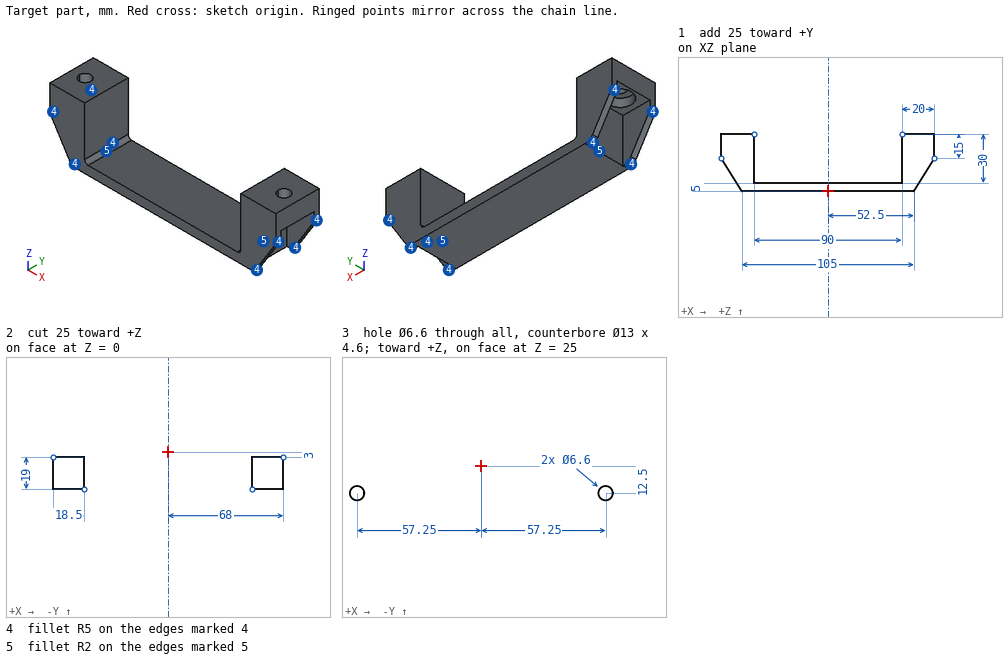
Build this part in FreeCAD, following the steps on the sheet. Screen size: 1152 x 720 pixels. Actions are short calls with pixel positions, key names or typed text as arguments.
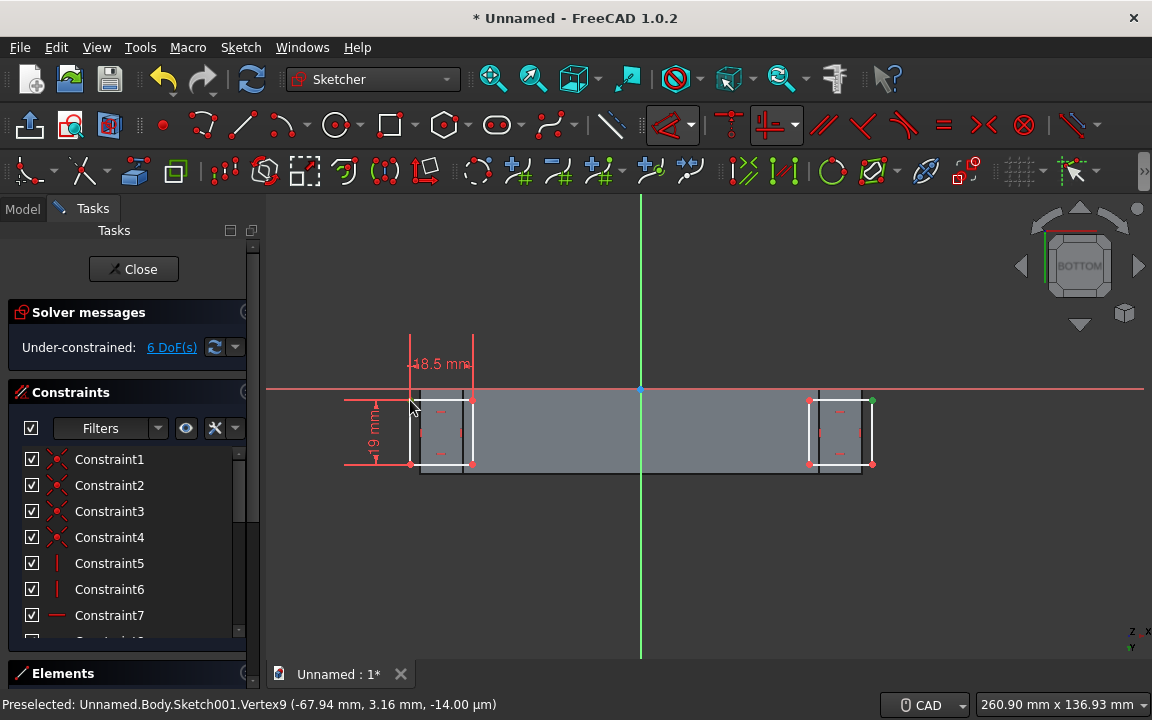
click(641, 602)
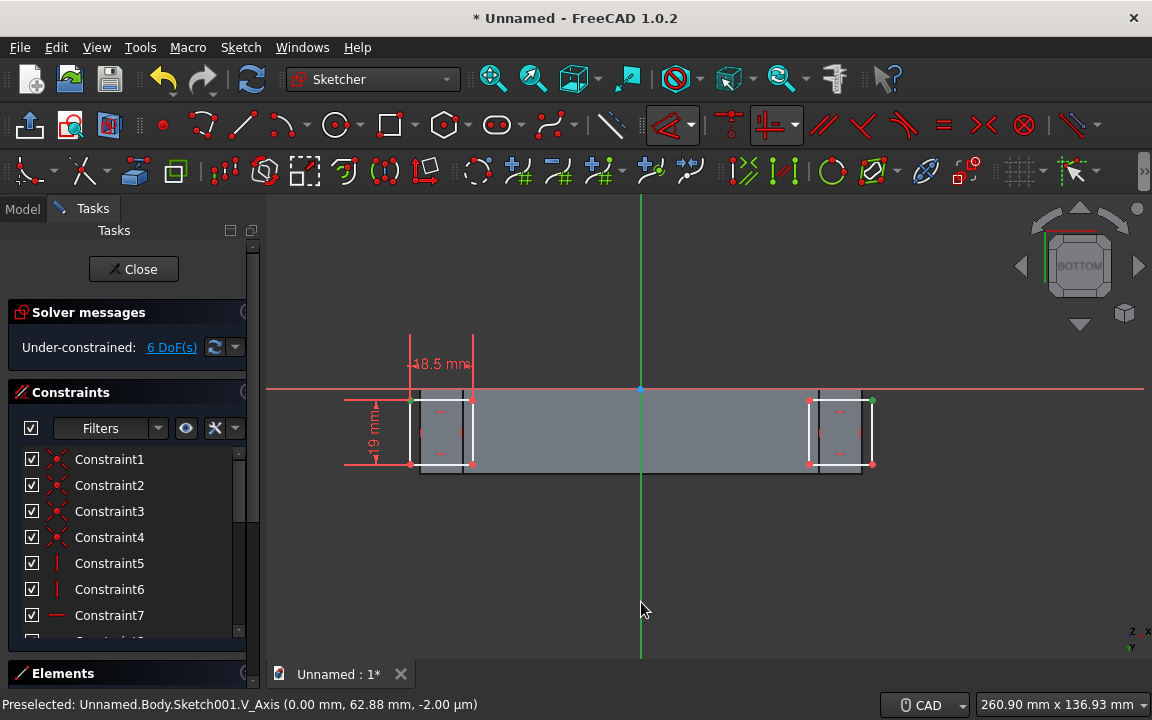
click(984, 126)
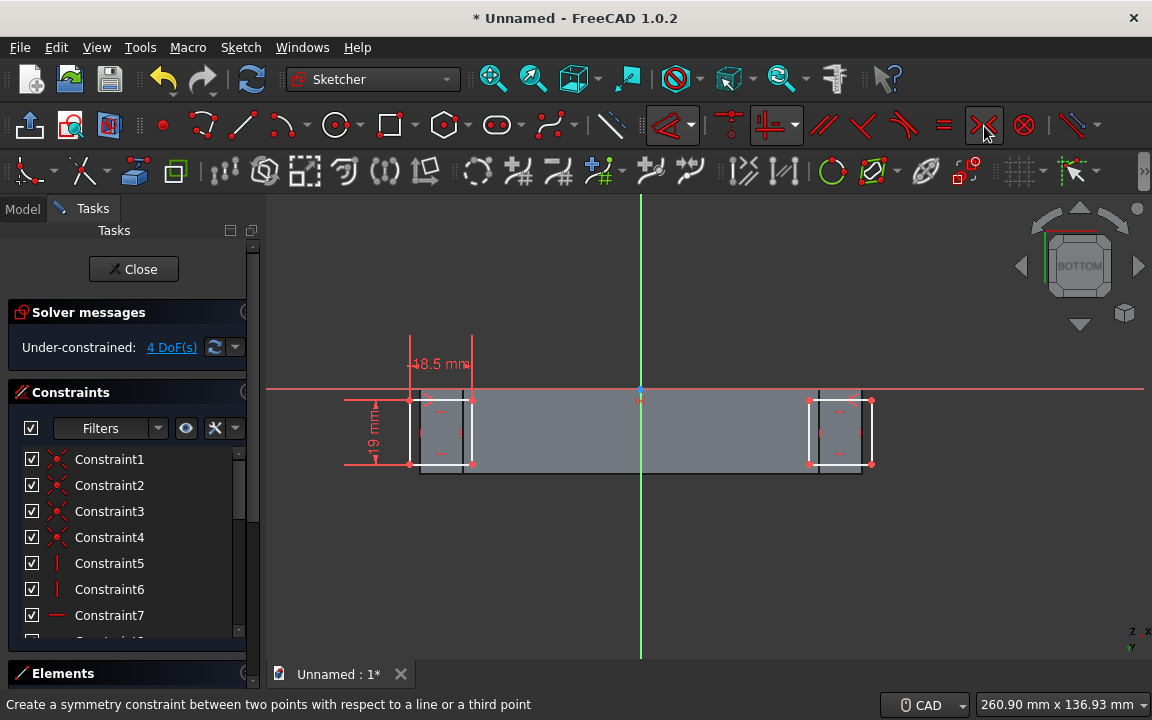
click(809, 465)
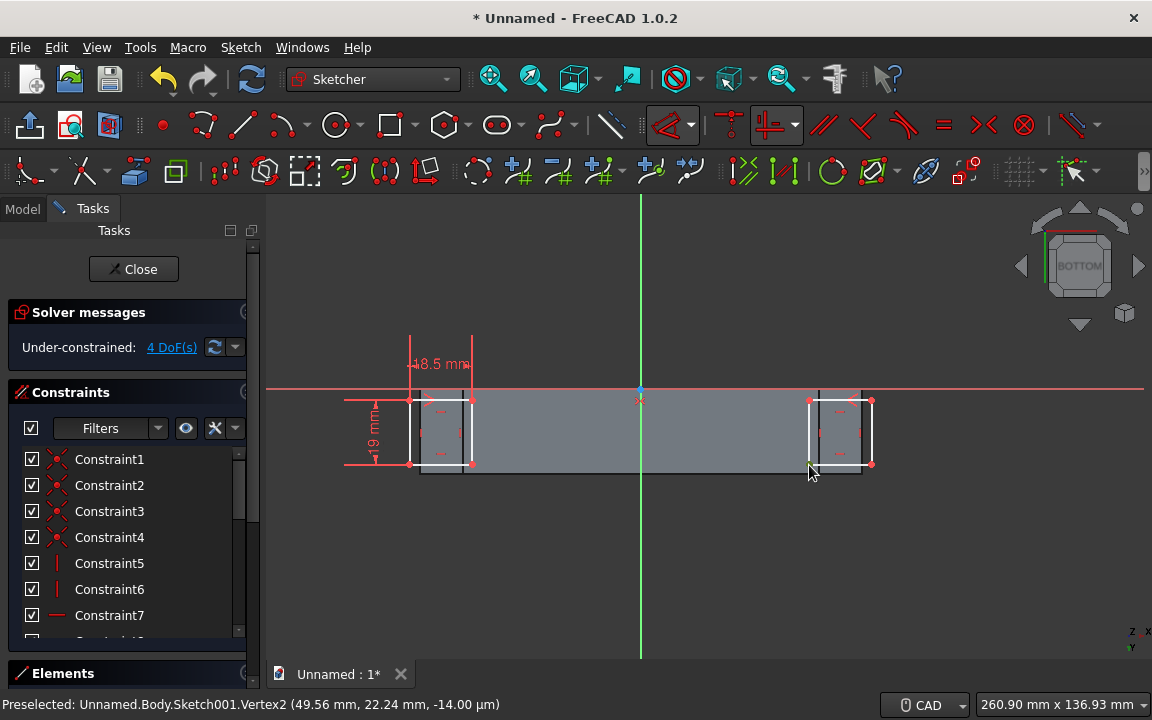
click(472, 465)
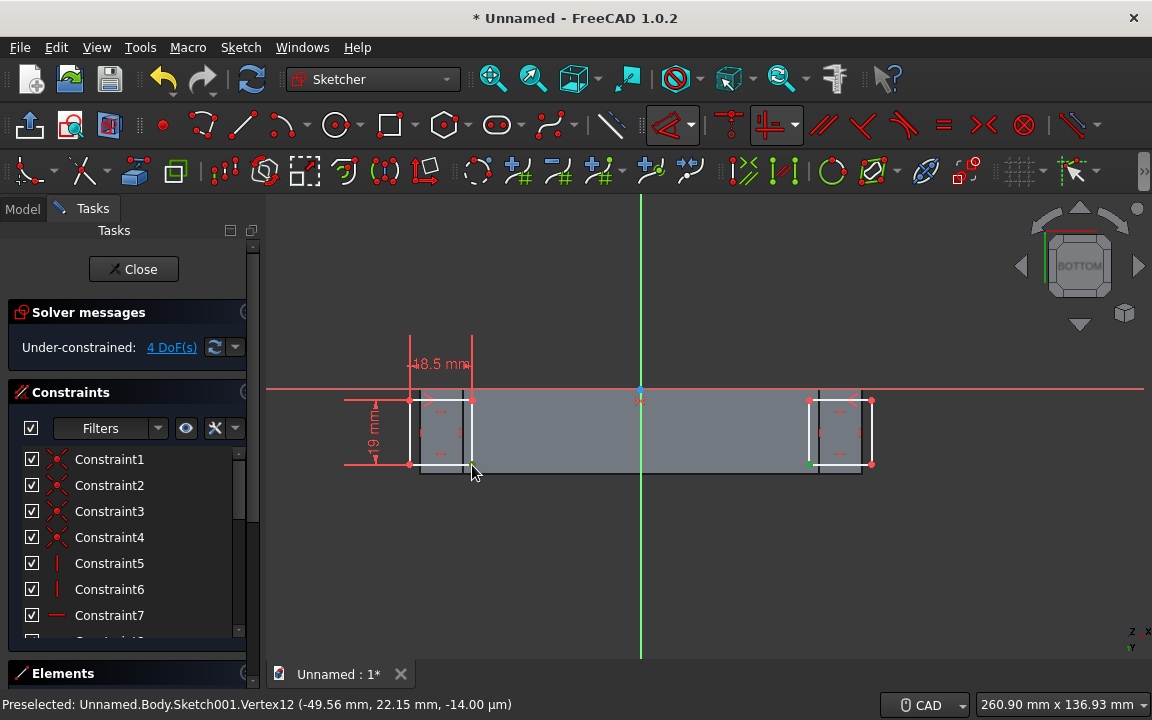
click(641, 602)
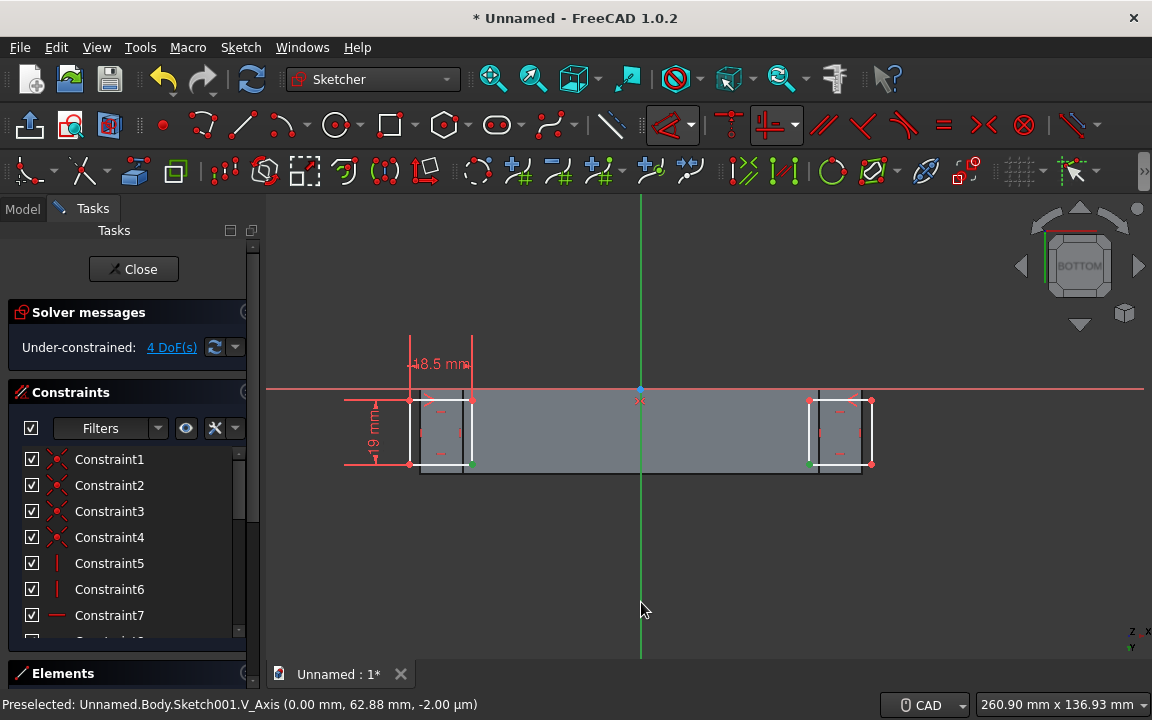
click(984, 126)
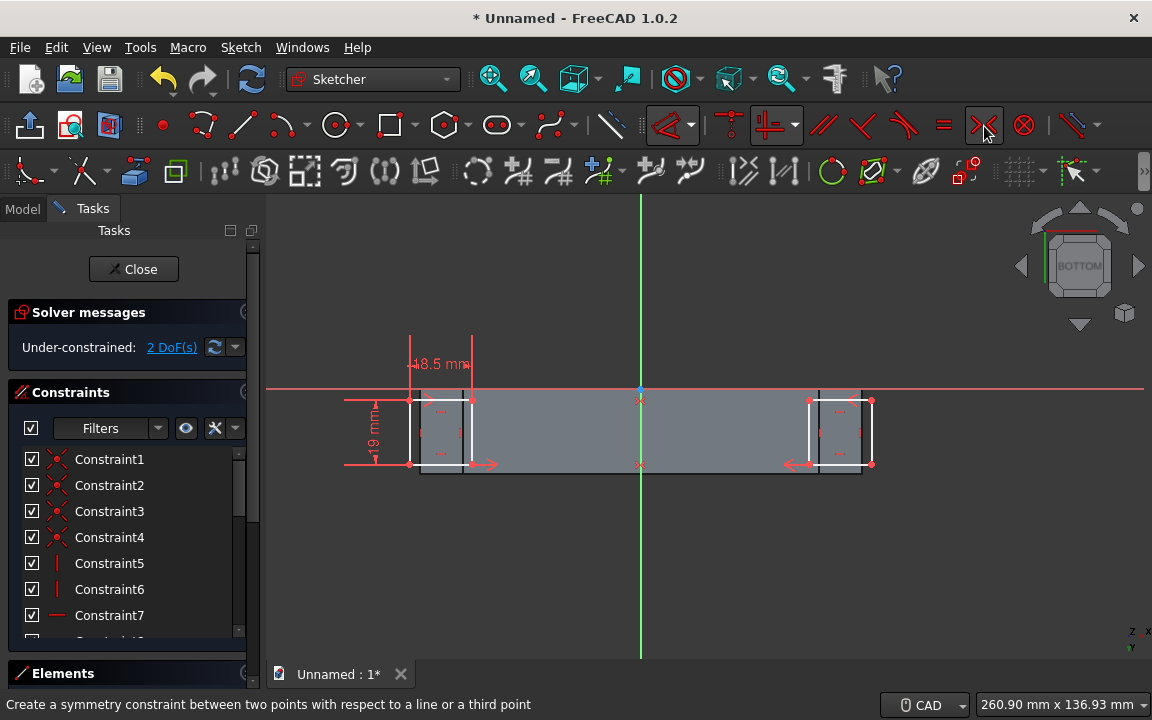
scroll(809, 400, up, 7)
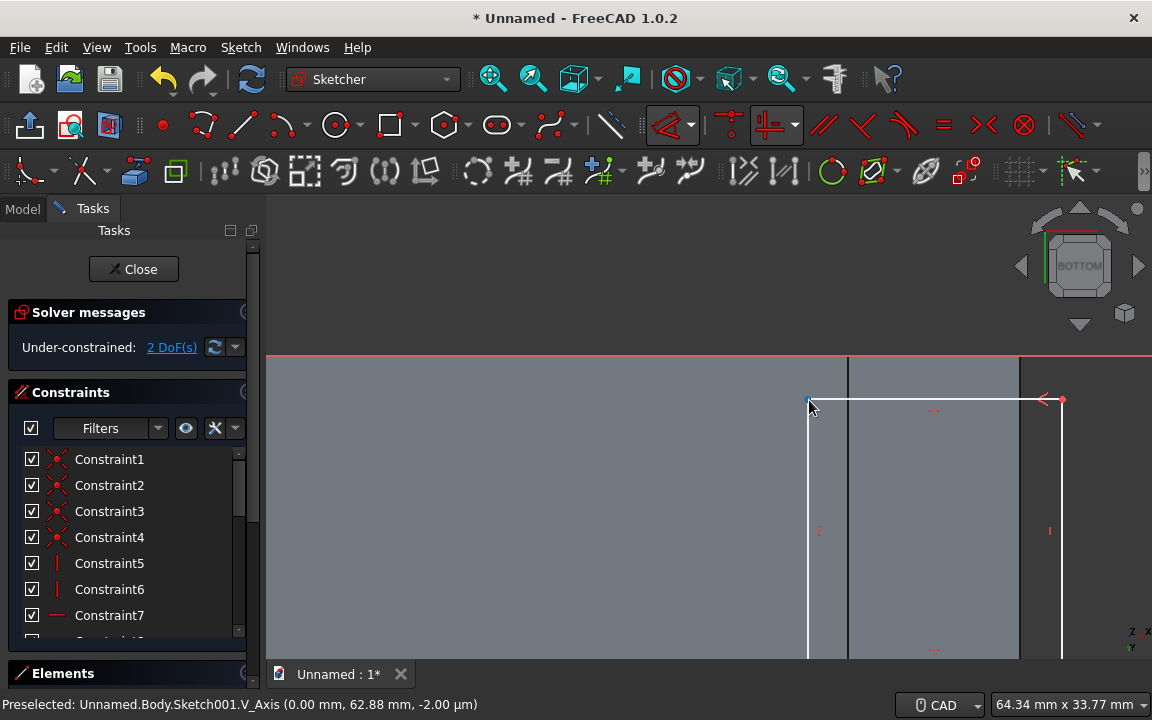
click(808, 399)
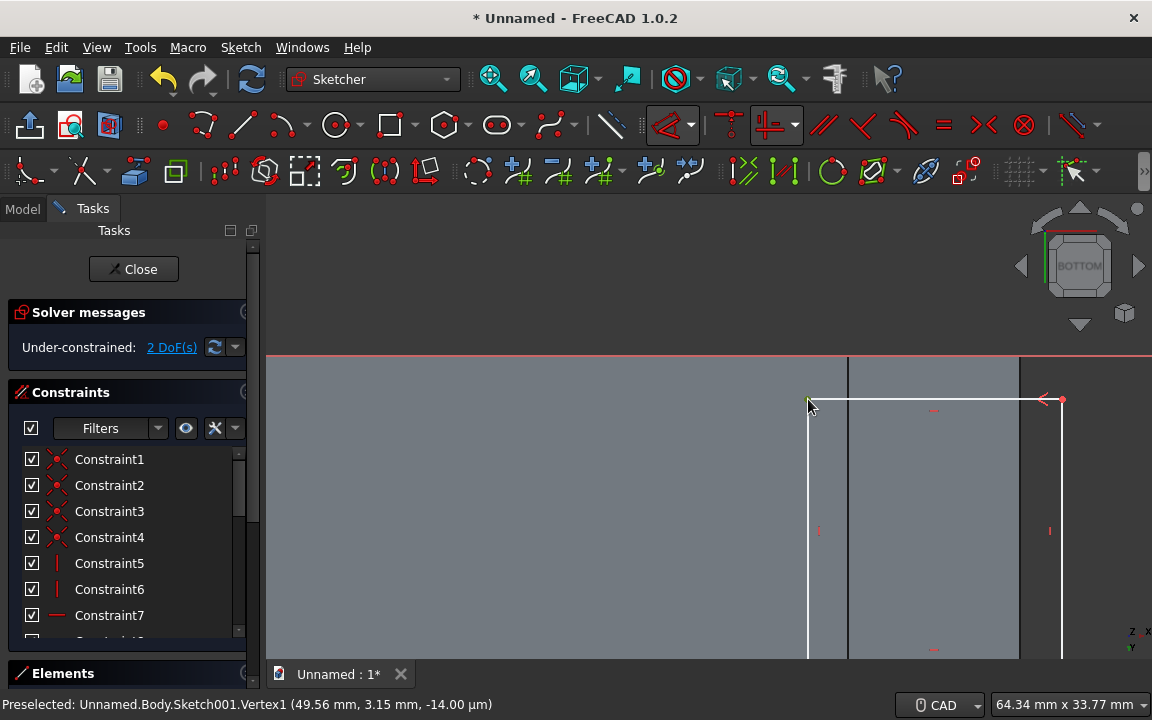
key(i)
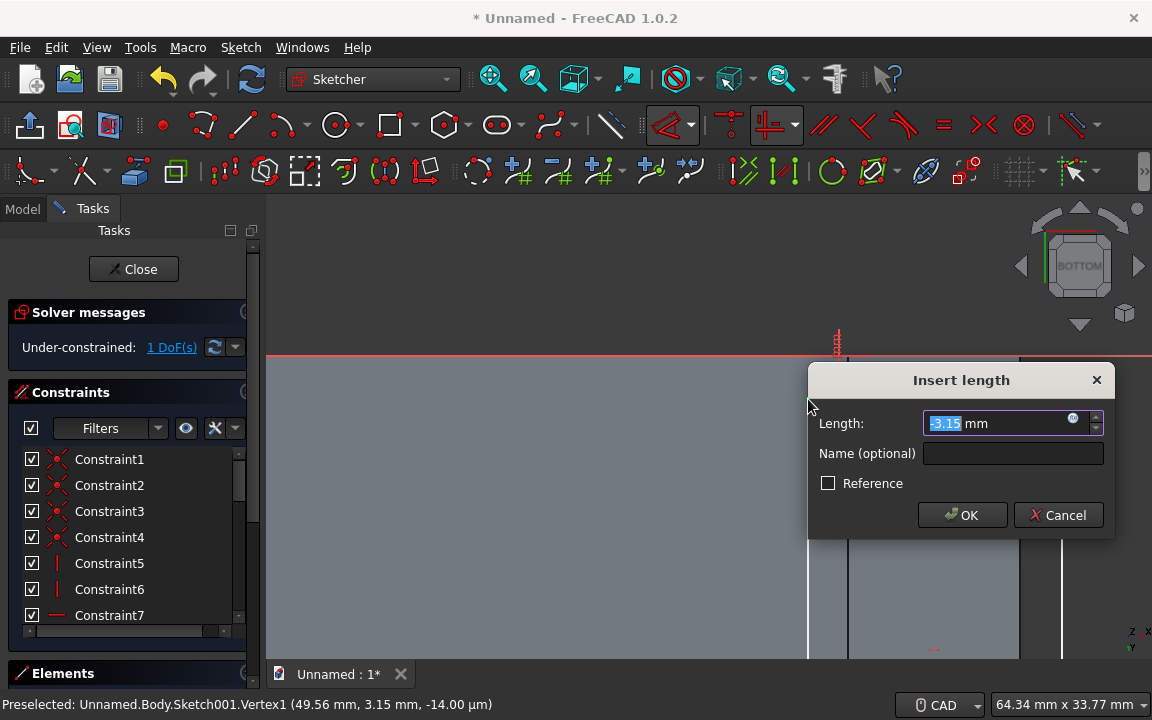
text(-3)
key(Return)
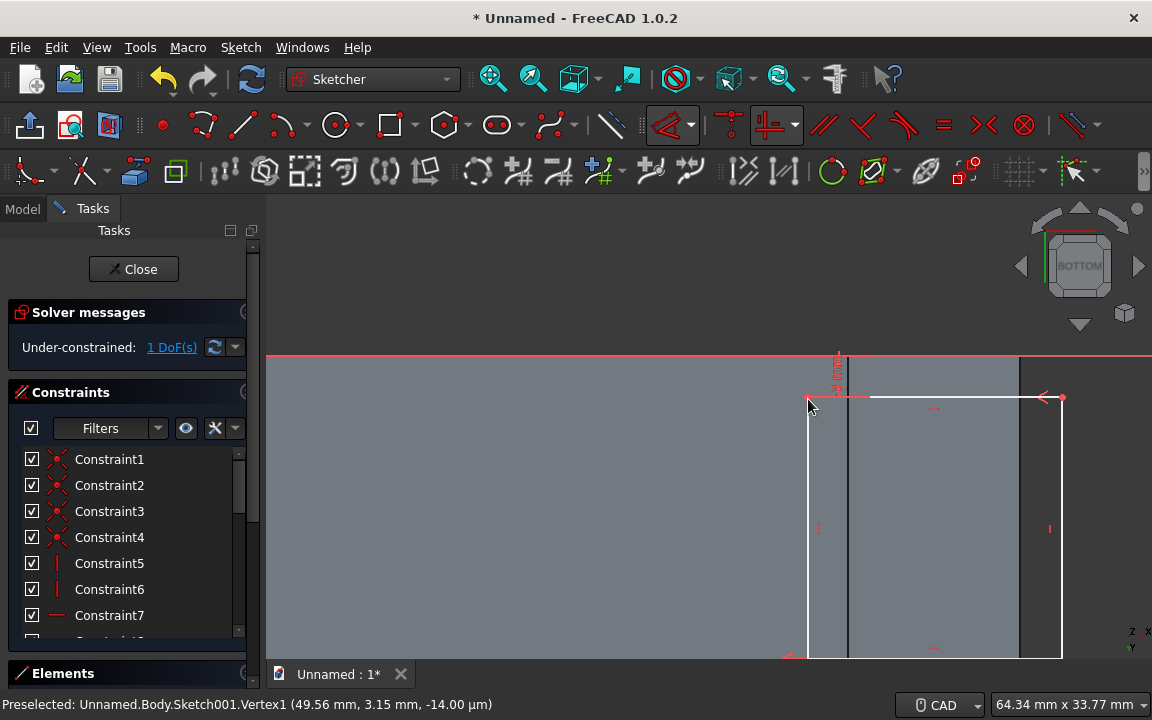
scroll(809, 400, down, 7)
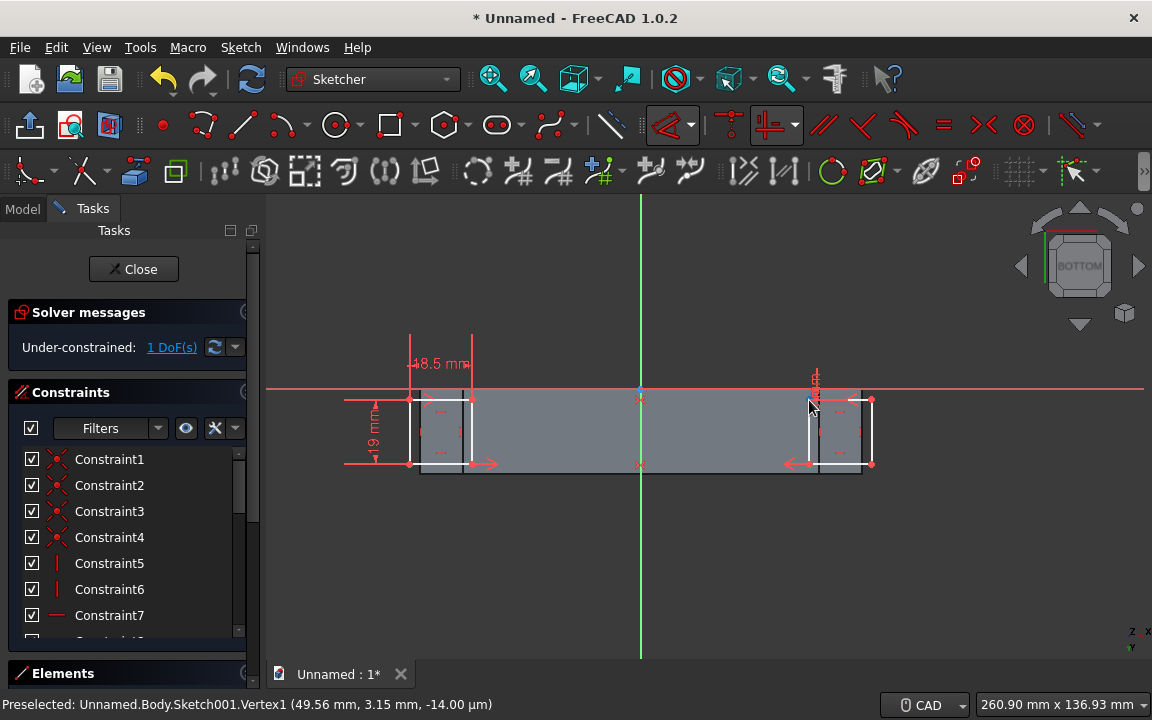
click(872, 464)